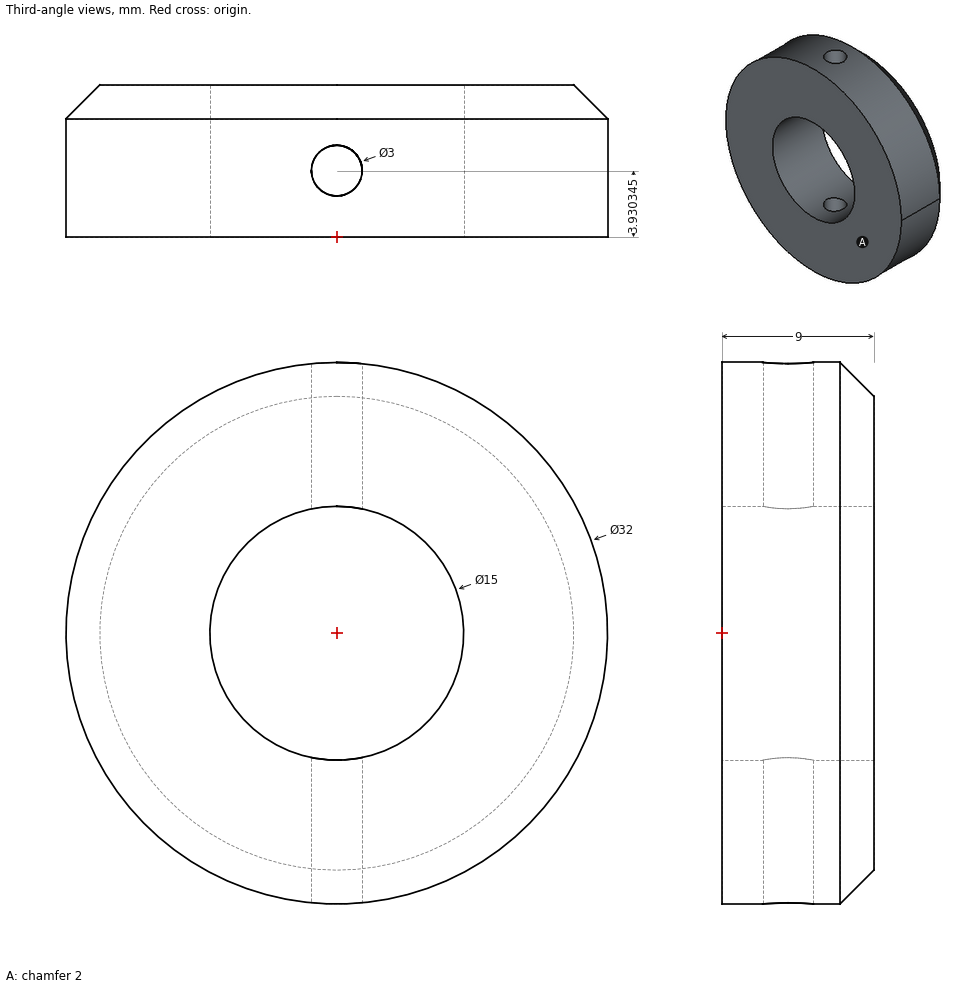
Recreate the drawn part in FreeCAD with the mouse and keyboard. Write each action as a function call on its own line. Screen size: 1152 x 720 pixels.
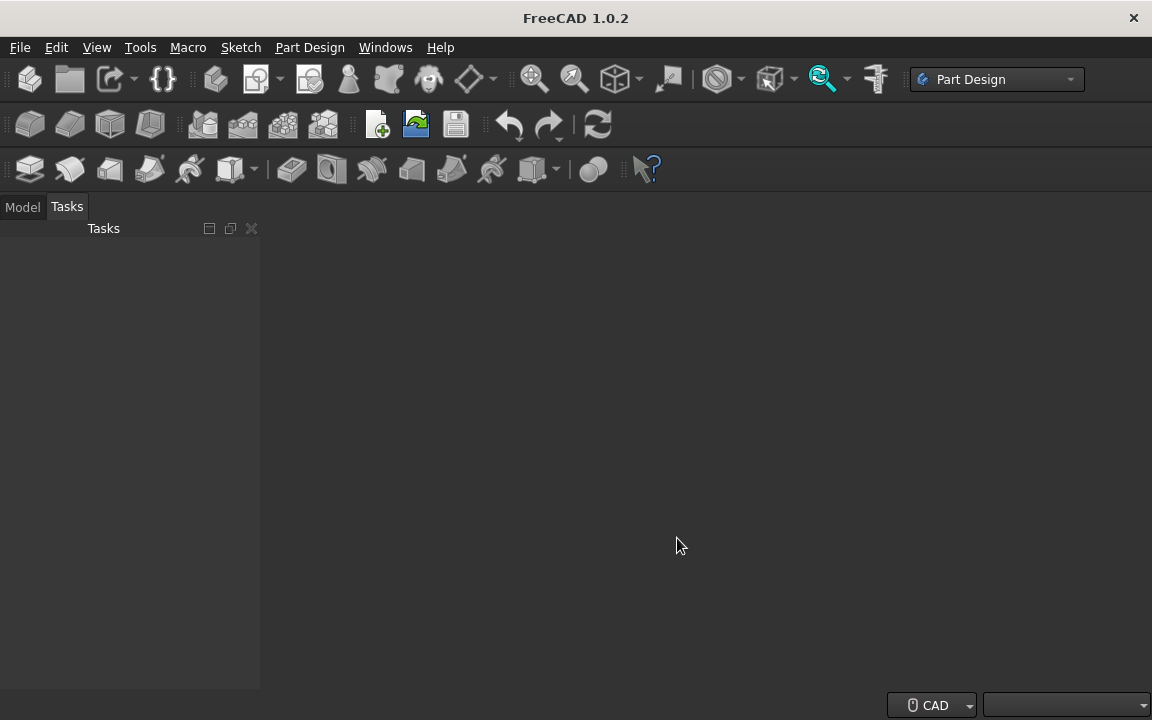
key(ctrl+n)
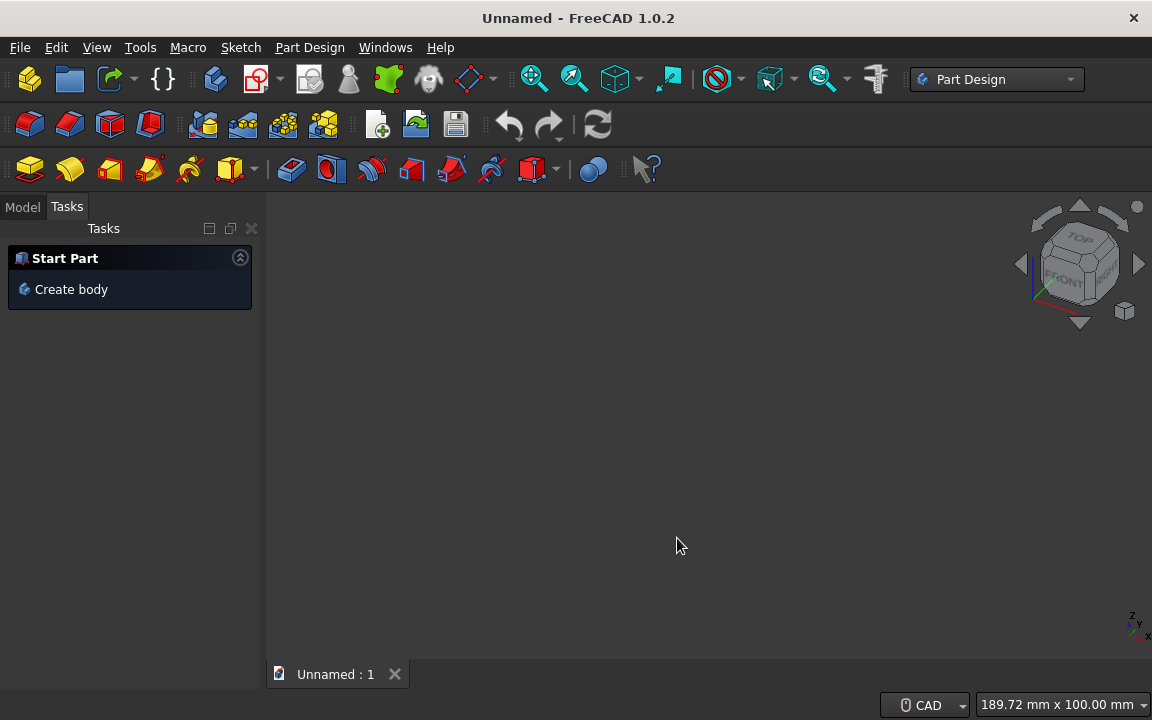
click(256, 80)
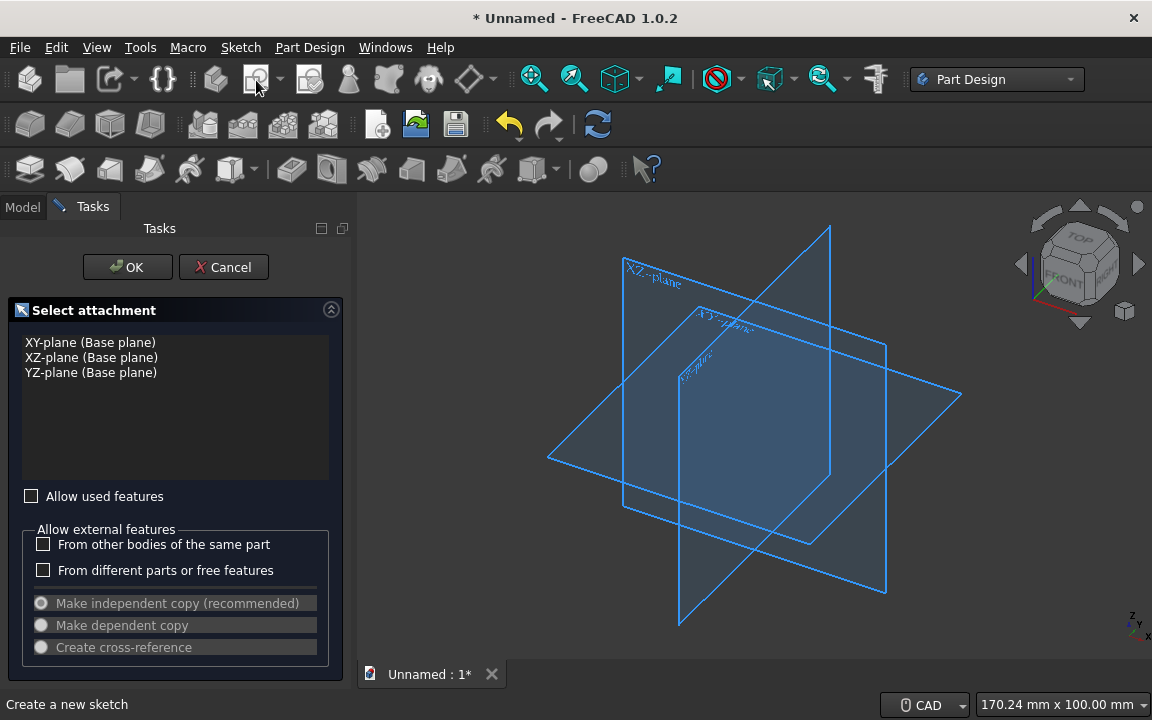
click(82, 358)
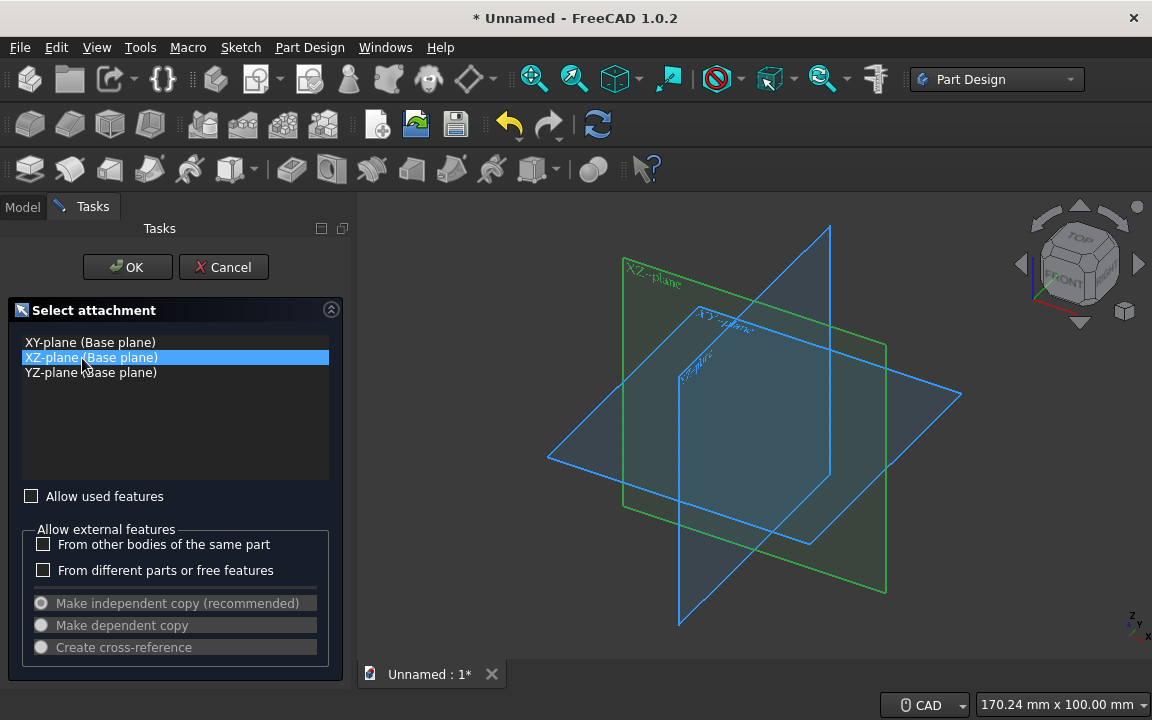
click(128, 267)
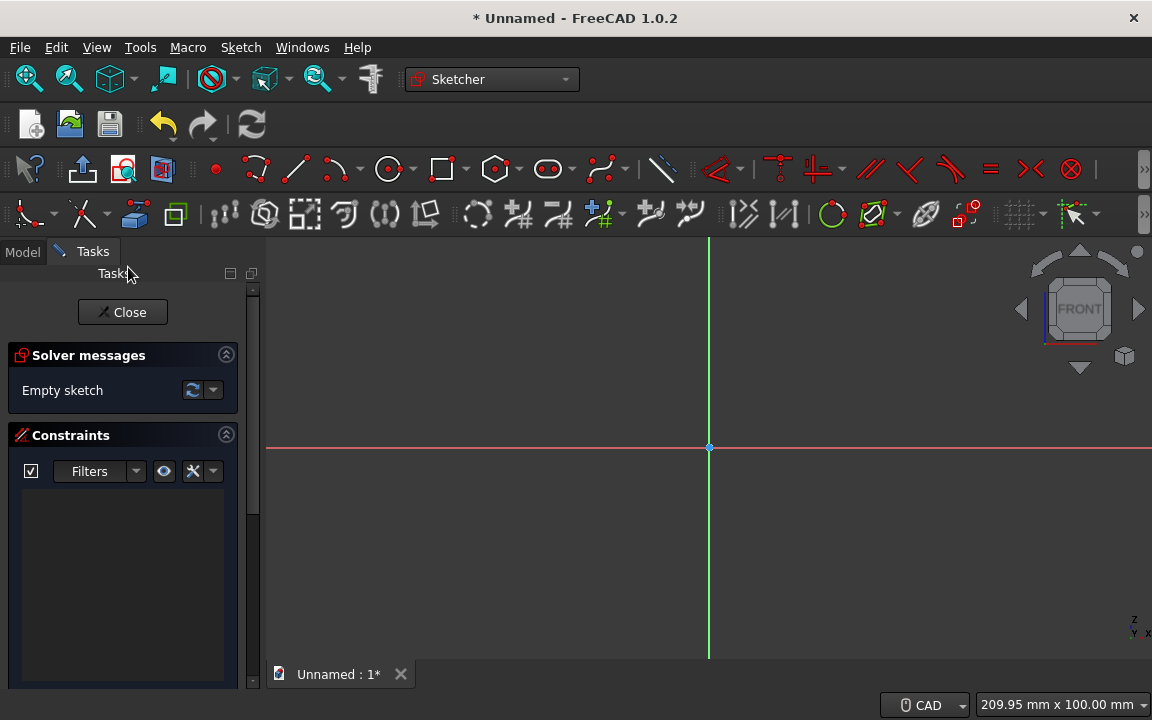
scroll(792, 448, up, 3)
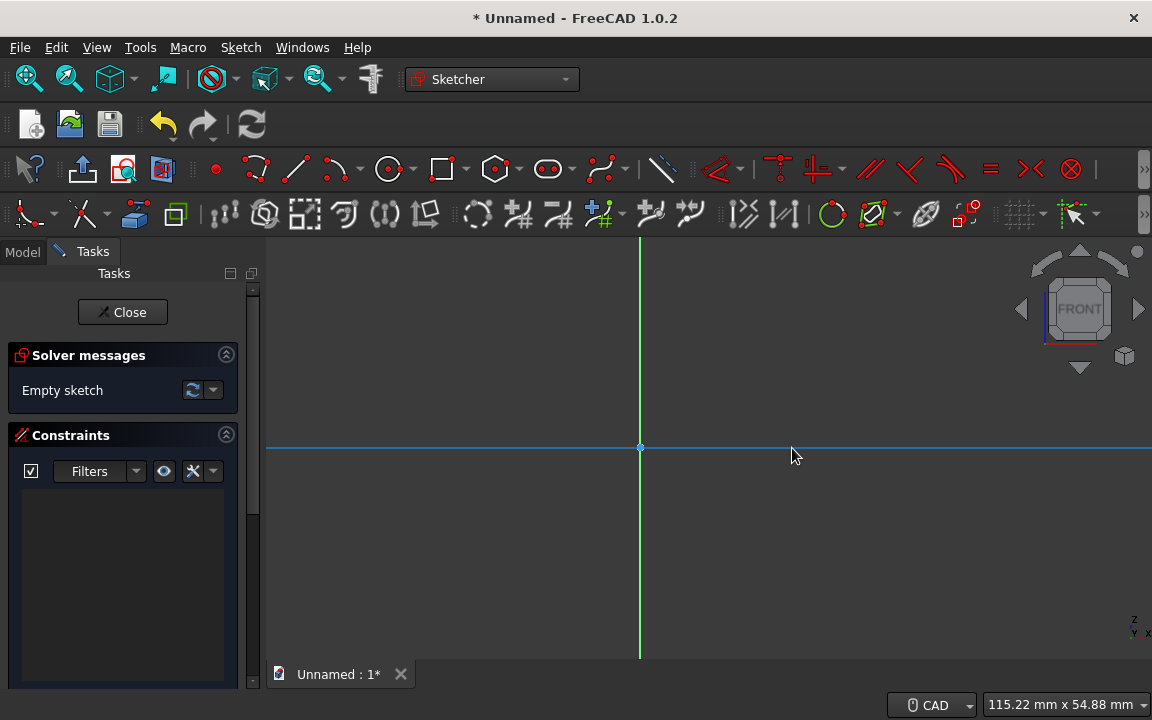
click(390, 170)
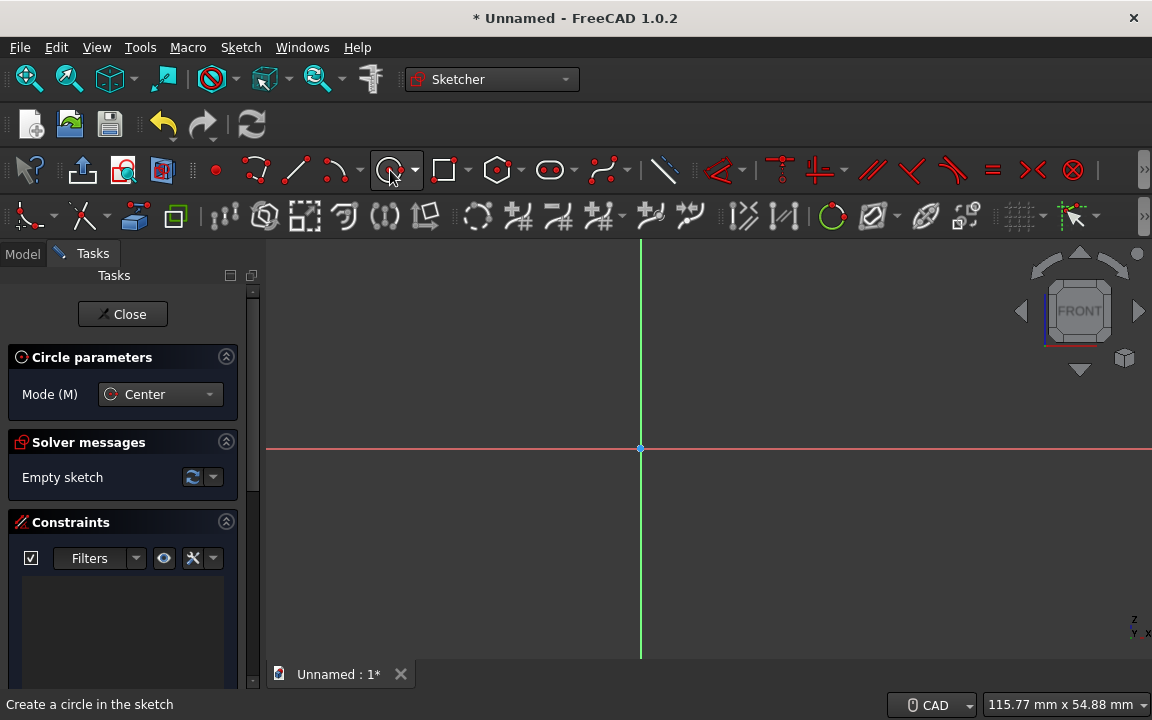
click(641, 449)
click(727, 362)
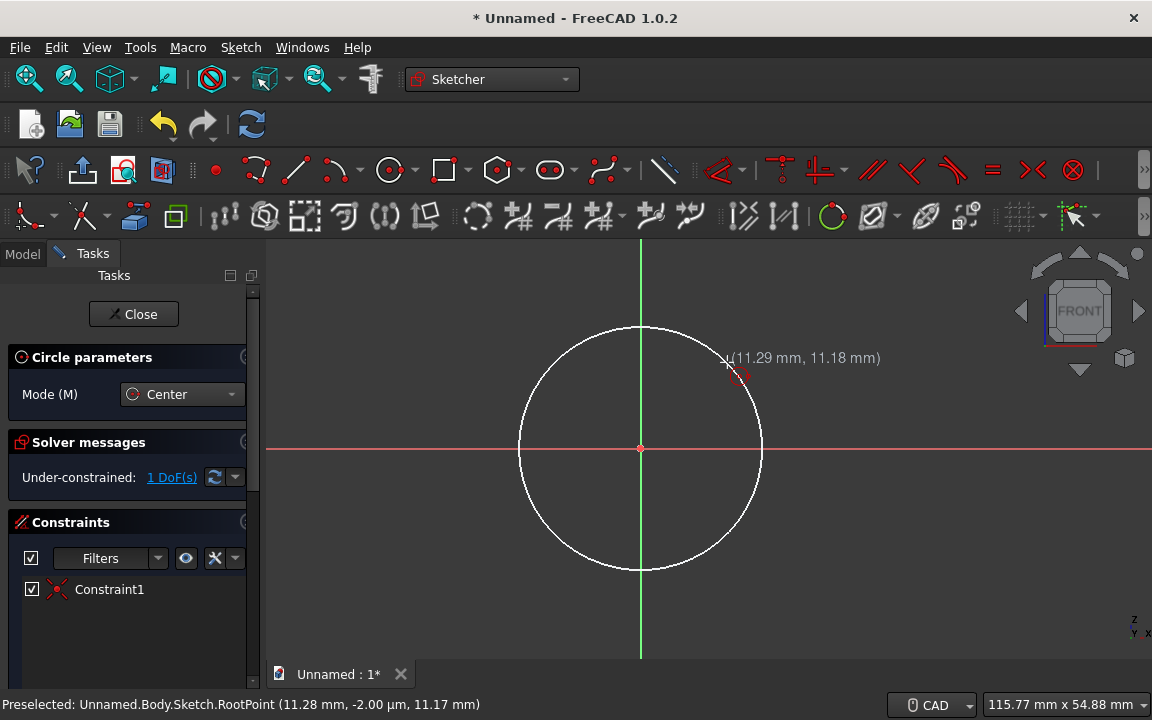
click(641, 449)
click(681, 408)
key(Escape)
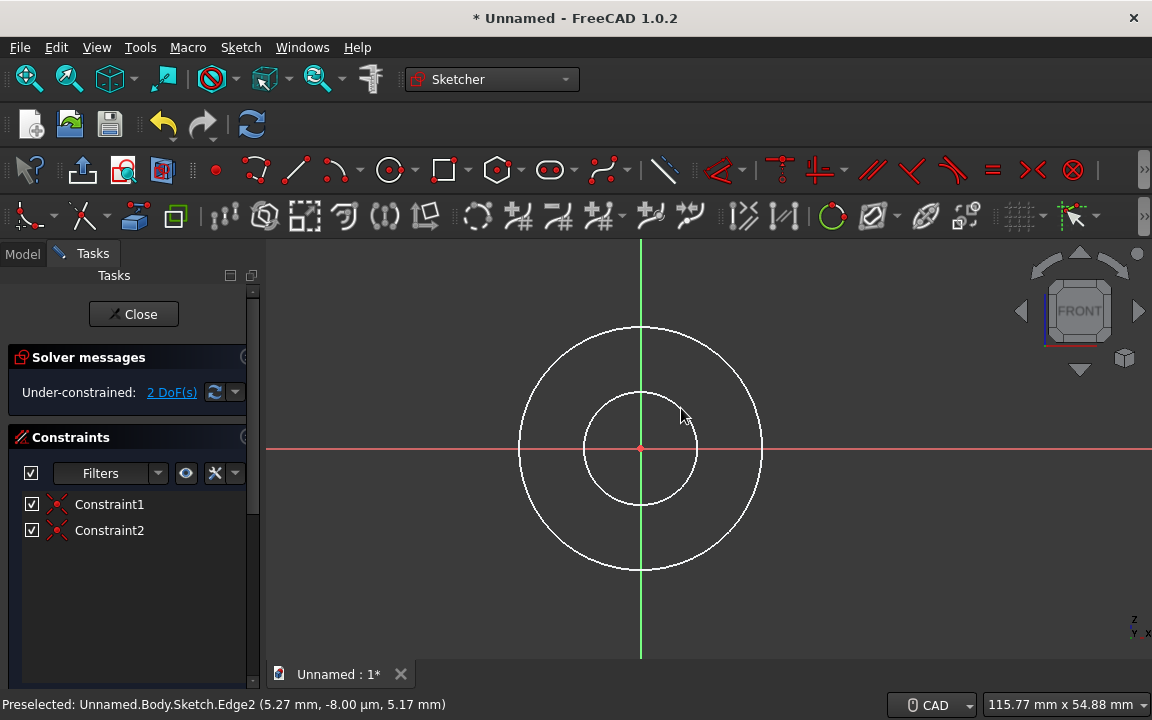
click(718, 170)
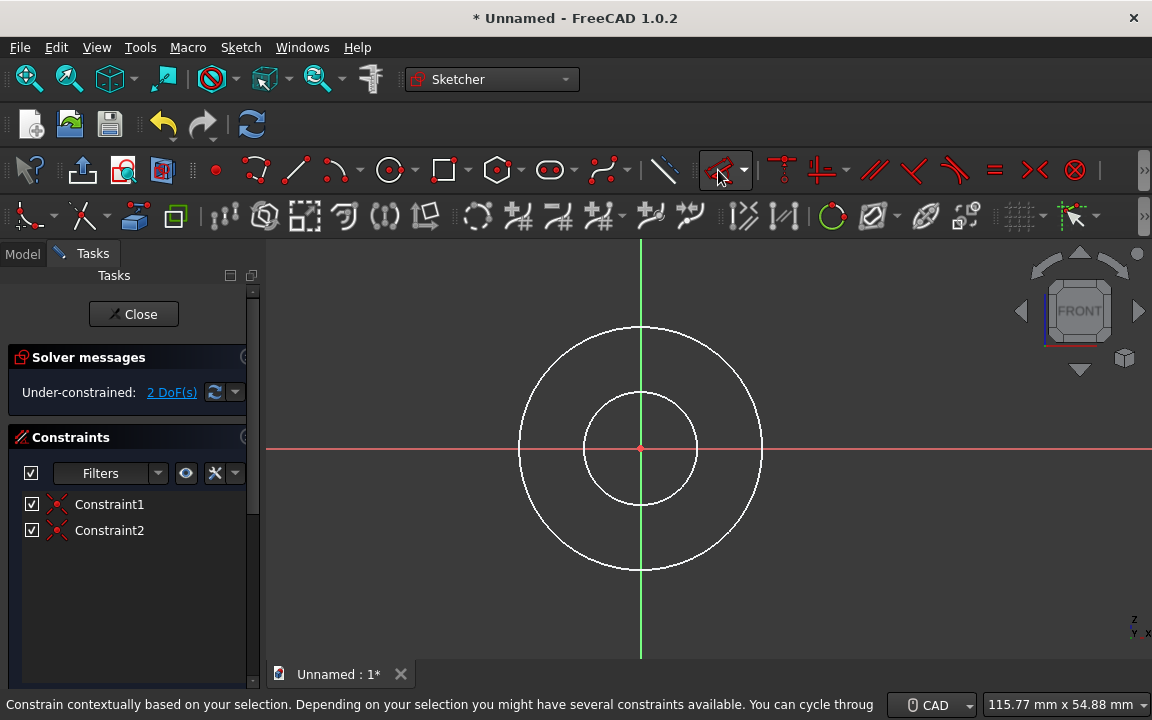
click(726, 362)
click(748, 339)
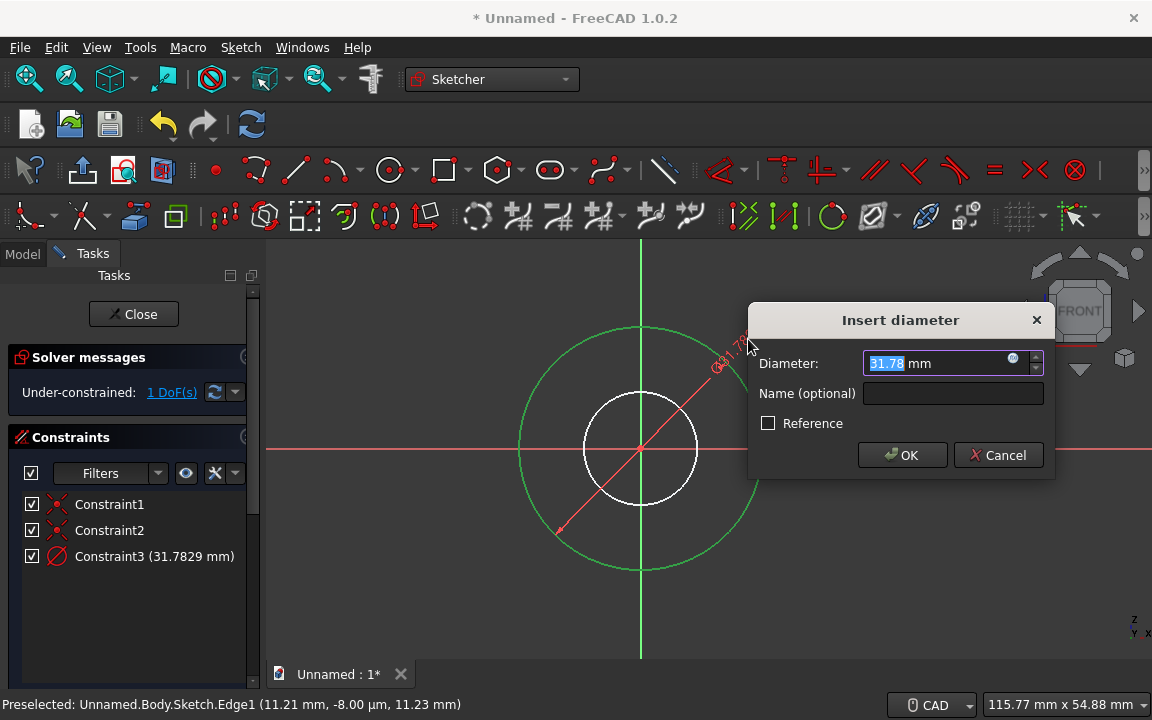
text(32)
key(Return)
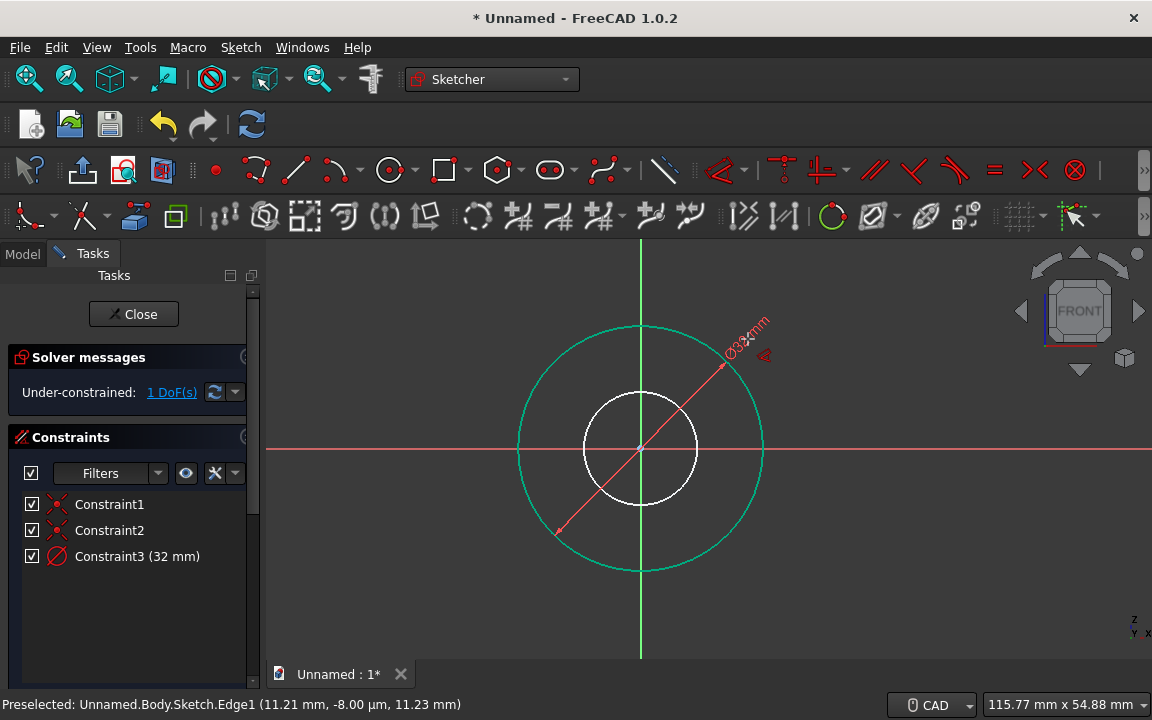
click(680, 408)
click(702, 385)